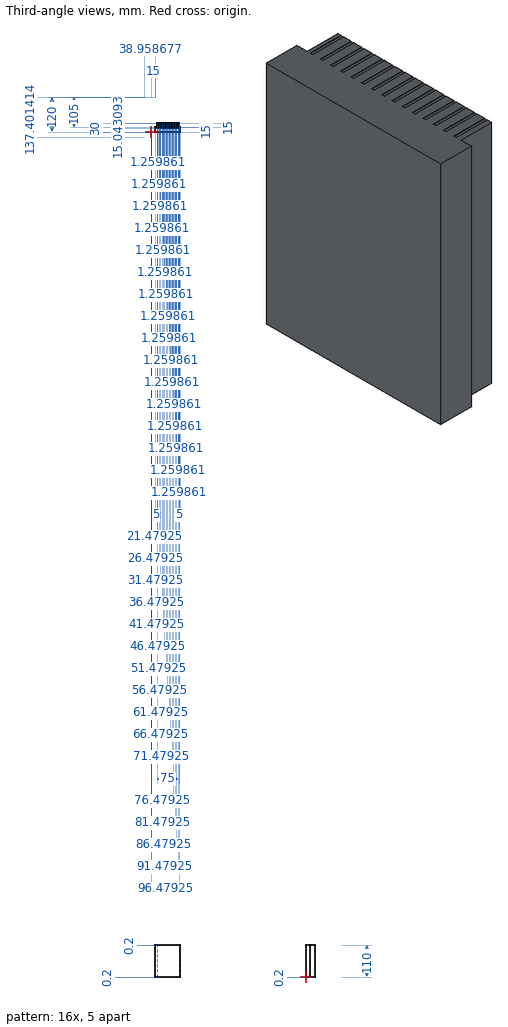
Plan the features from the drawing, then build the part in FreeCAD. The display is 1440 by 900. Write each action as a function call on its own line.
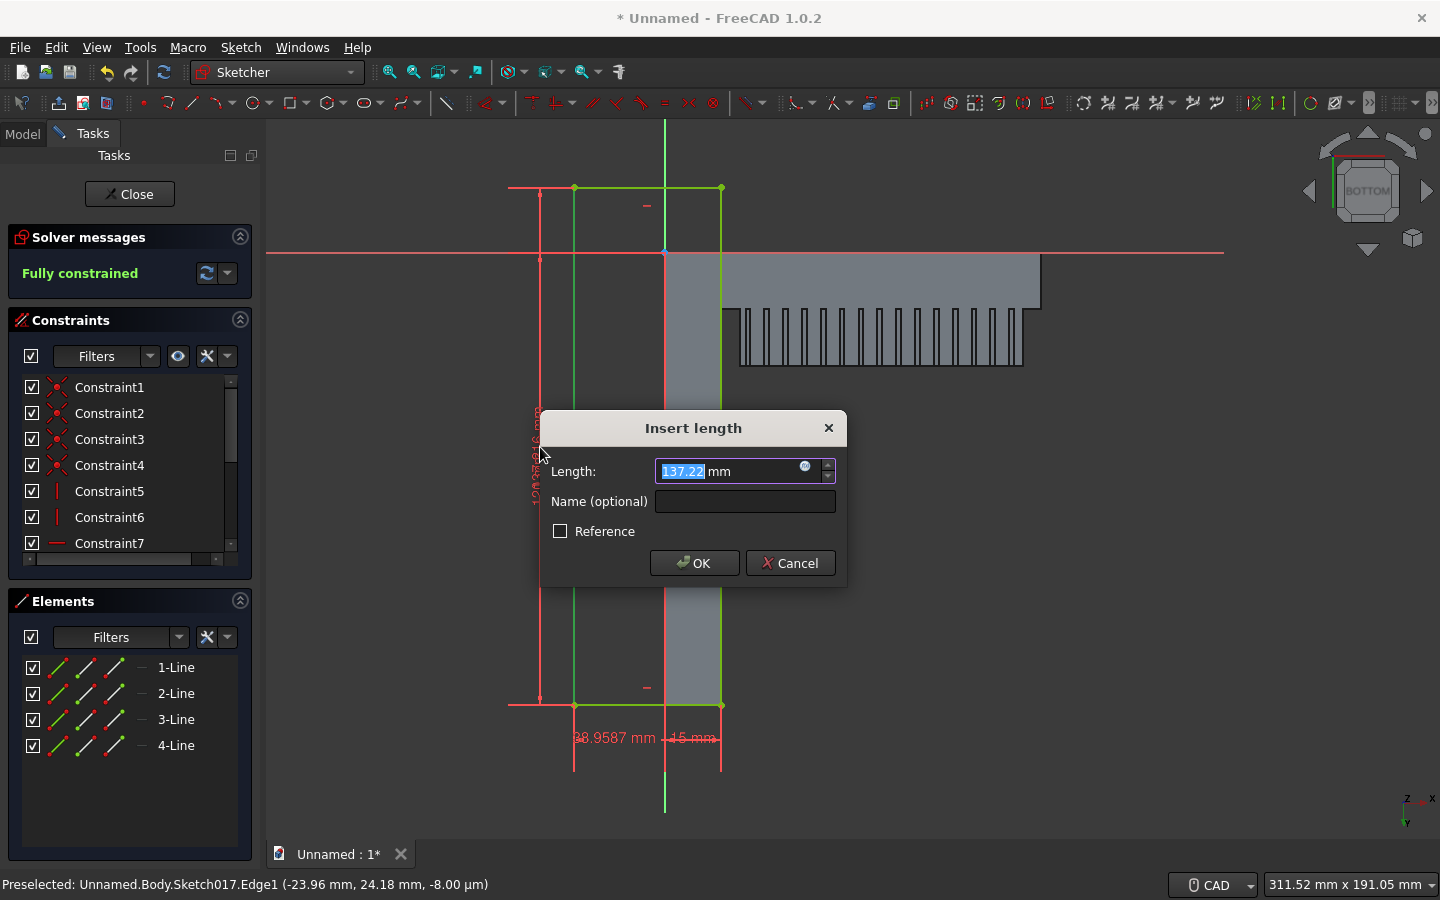
text(137.401414)
key(Return)
key(Escape)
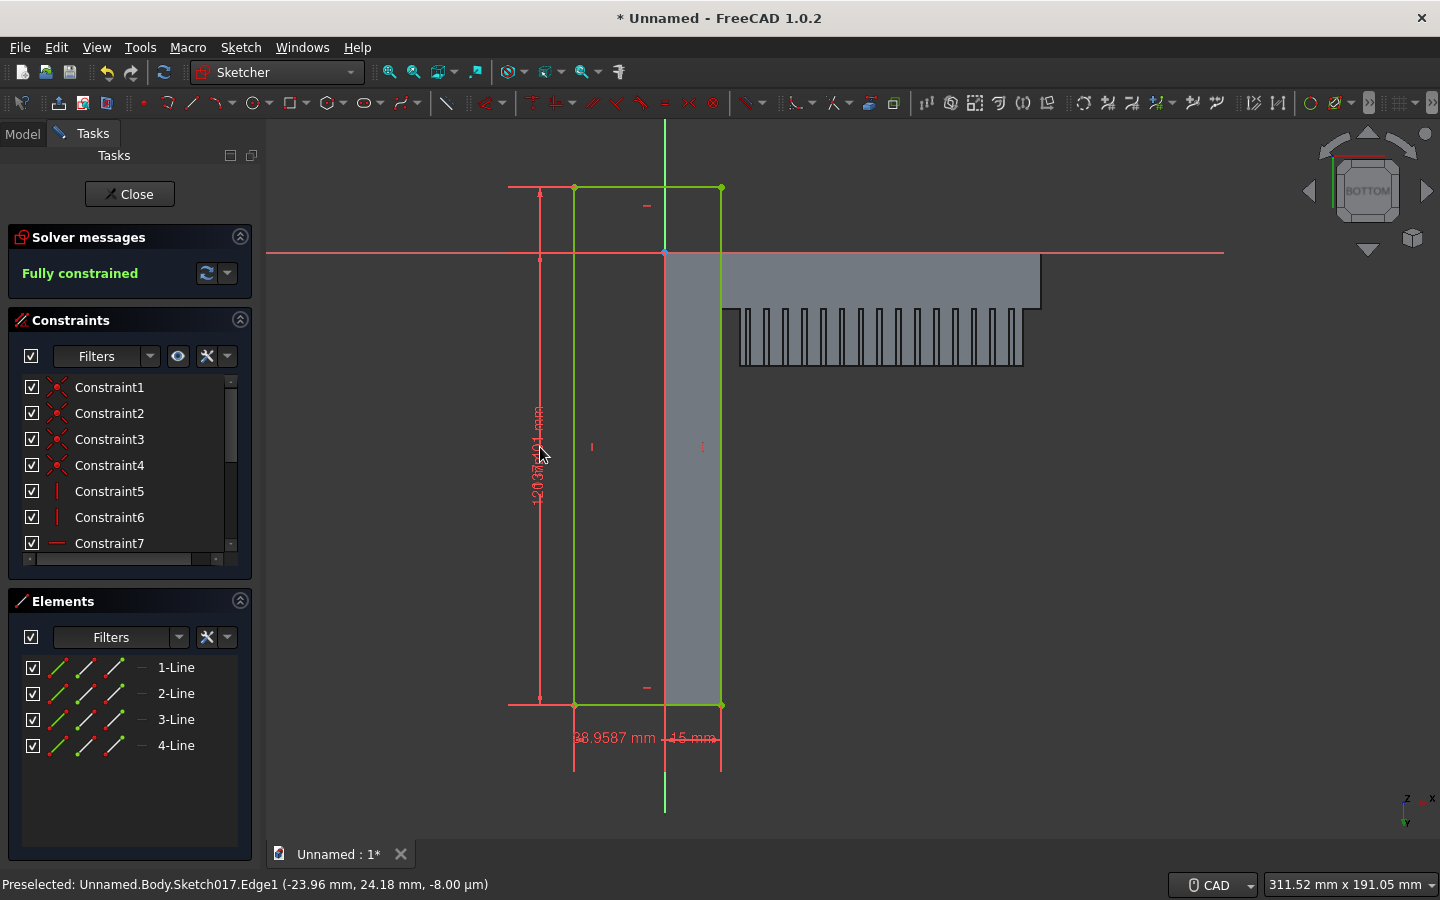
click(130, 194)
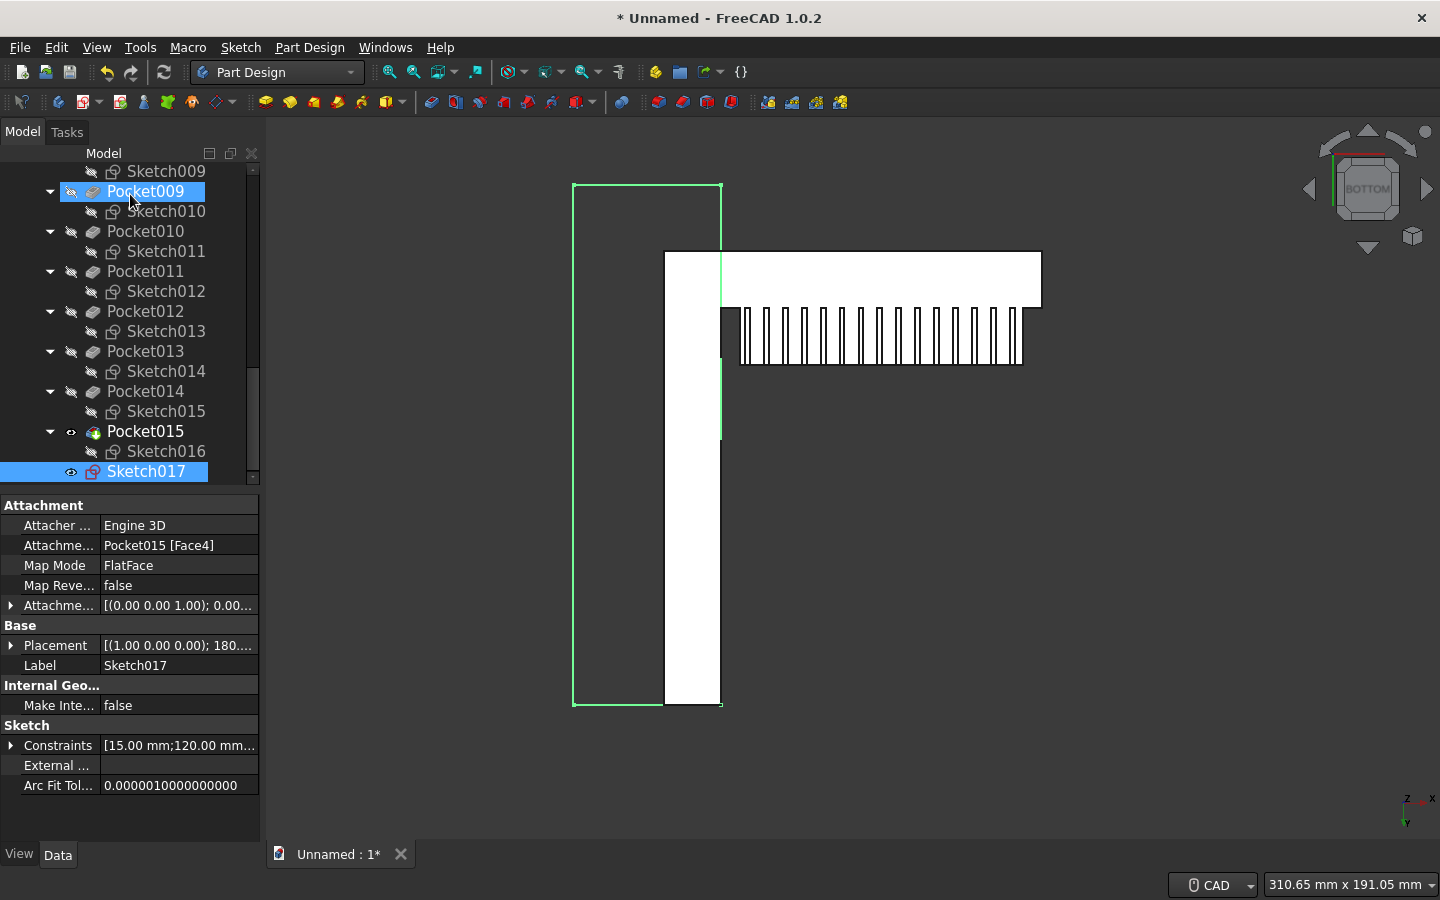
click(432, 102)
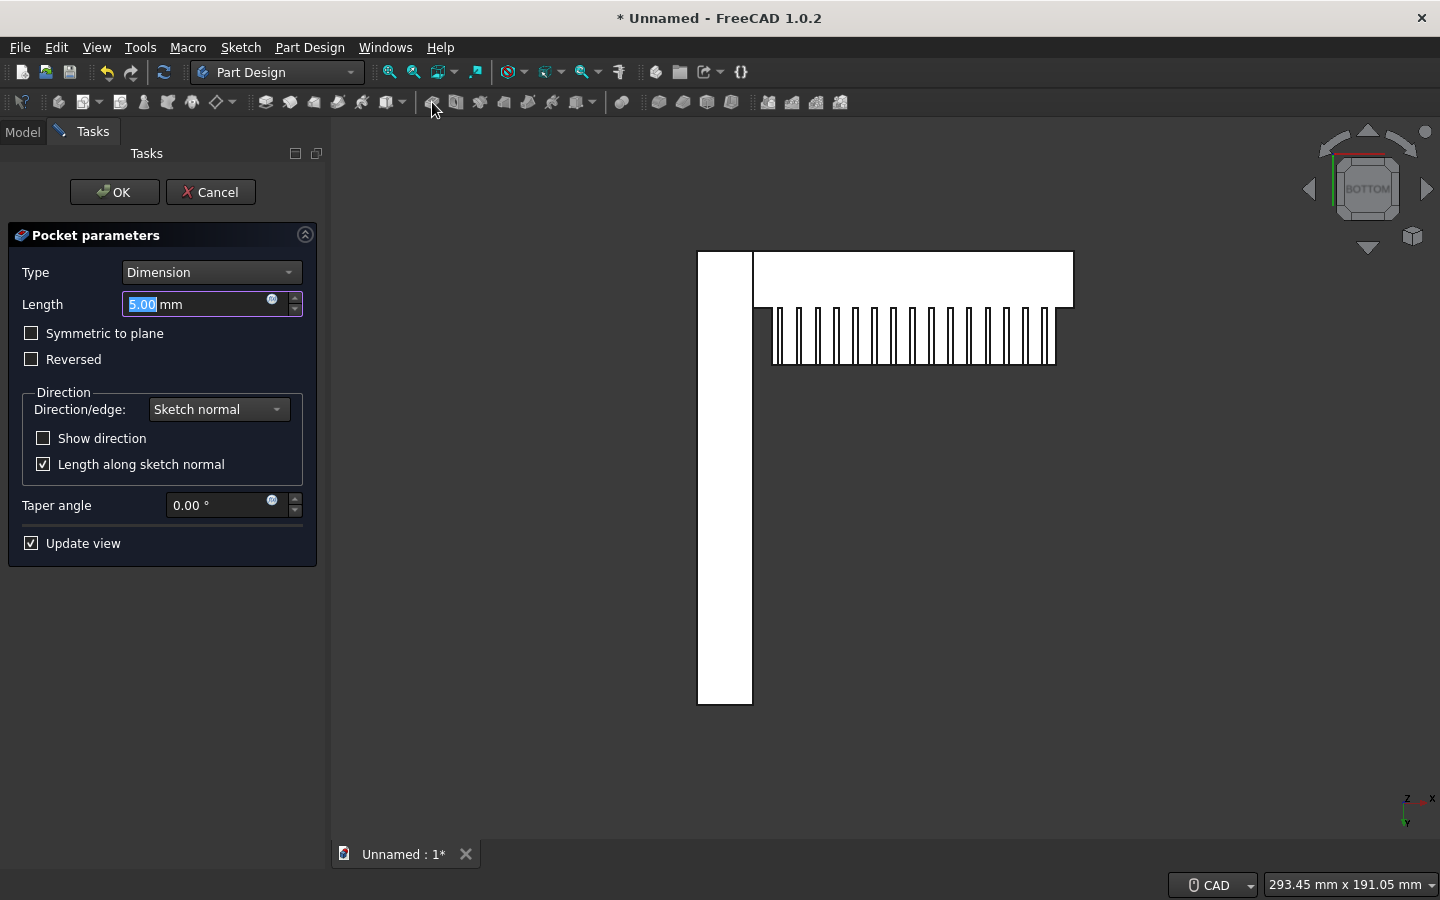
click(212, 272)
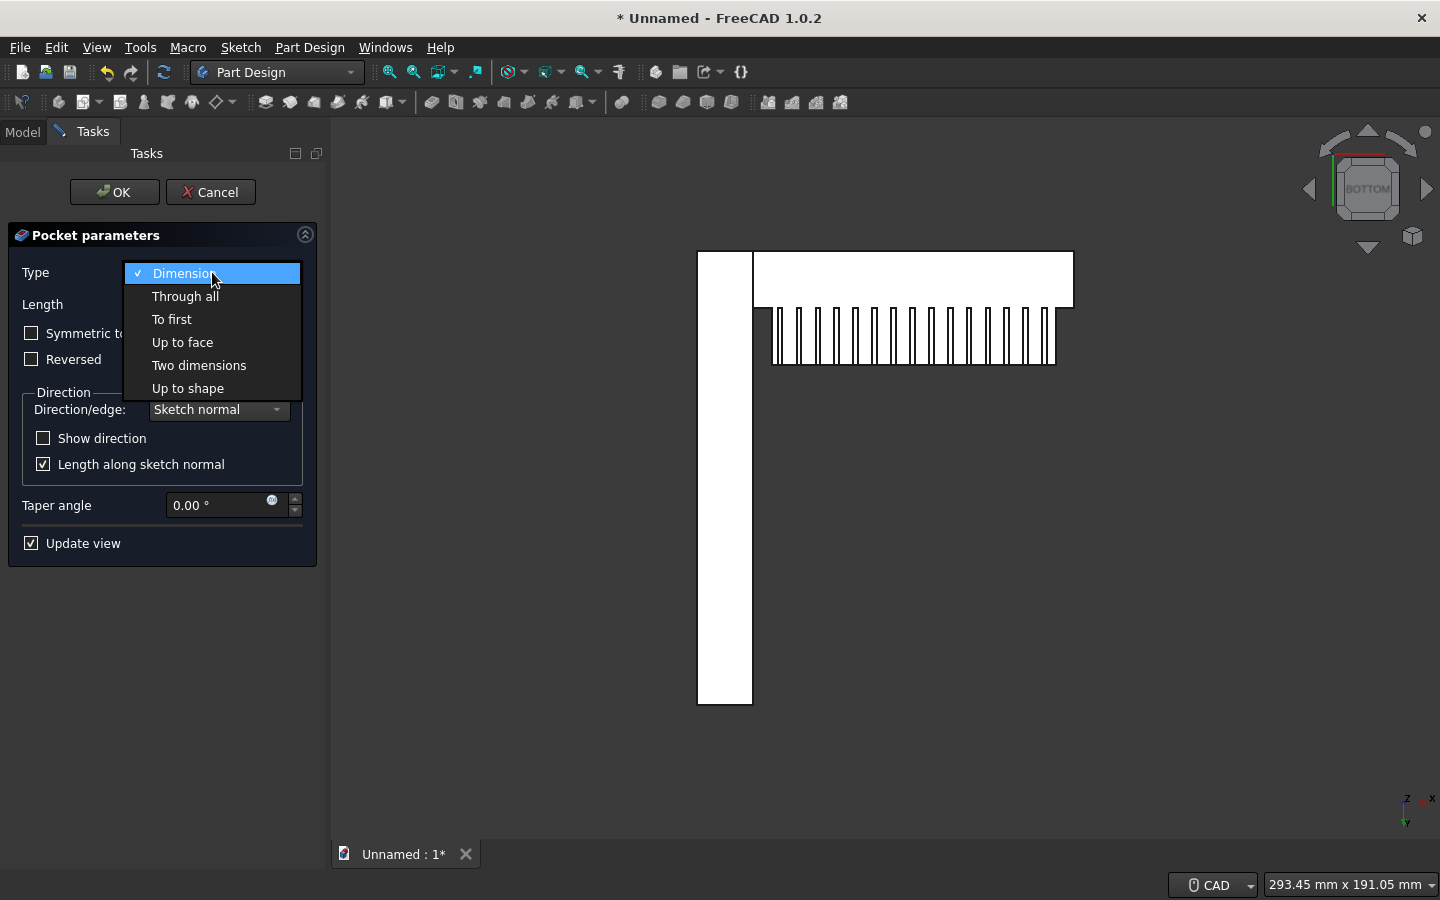
click(212, 296)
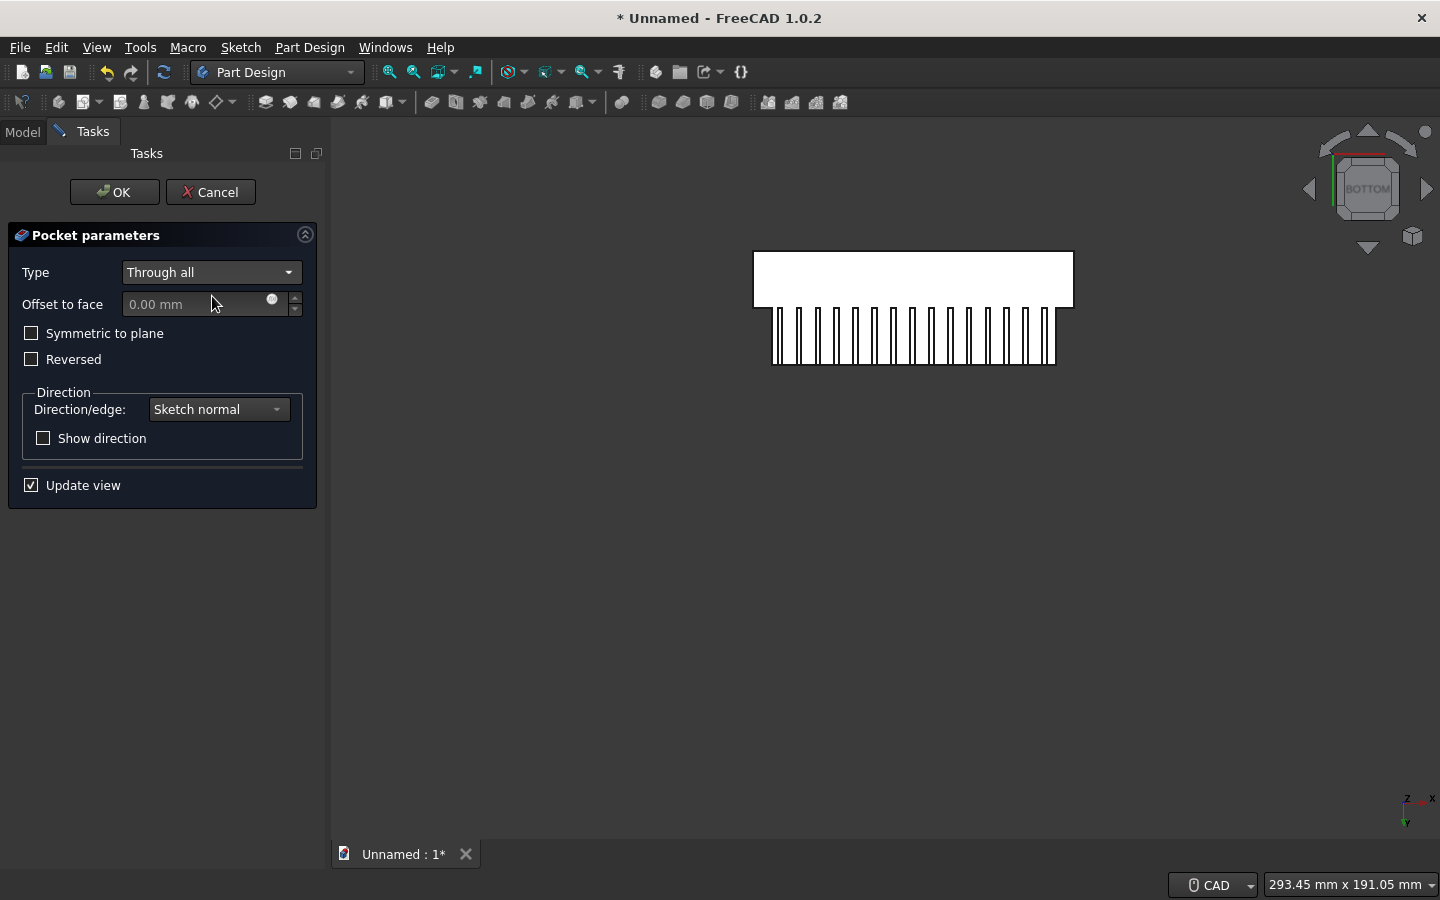
click(115, 192)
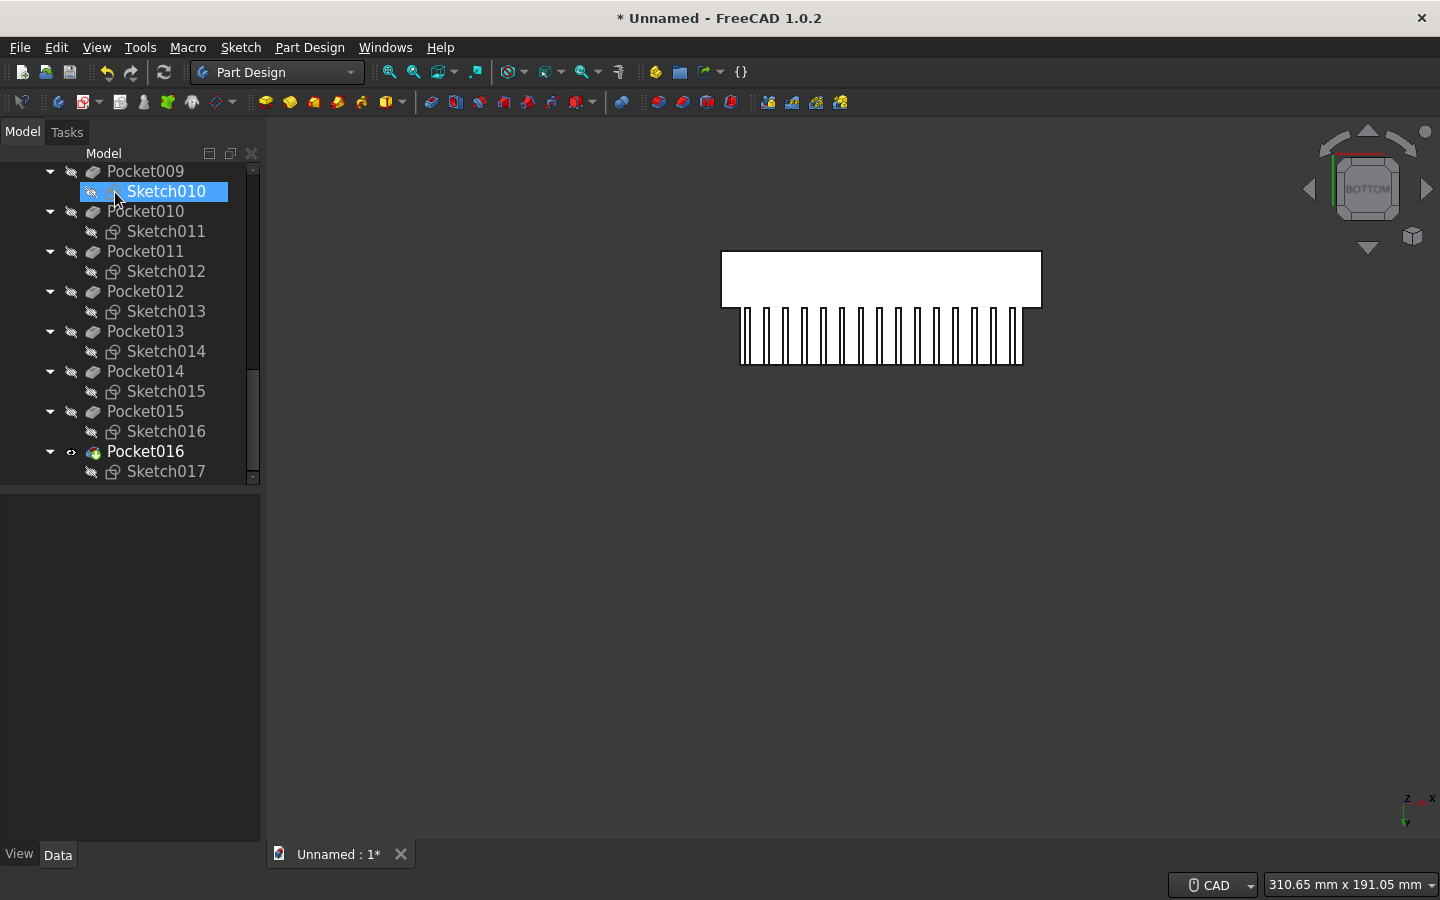
key(0)